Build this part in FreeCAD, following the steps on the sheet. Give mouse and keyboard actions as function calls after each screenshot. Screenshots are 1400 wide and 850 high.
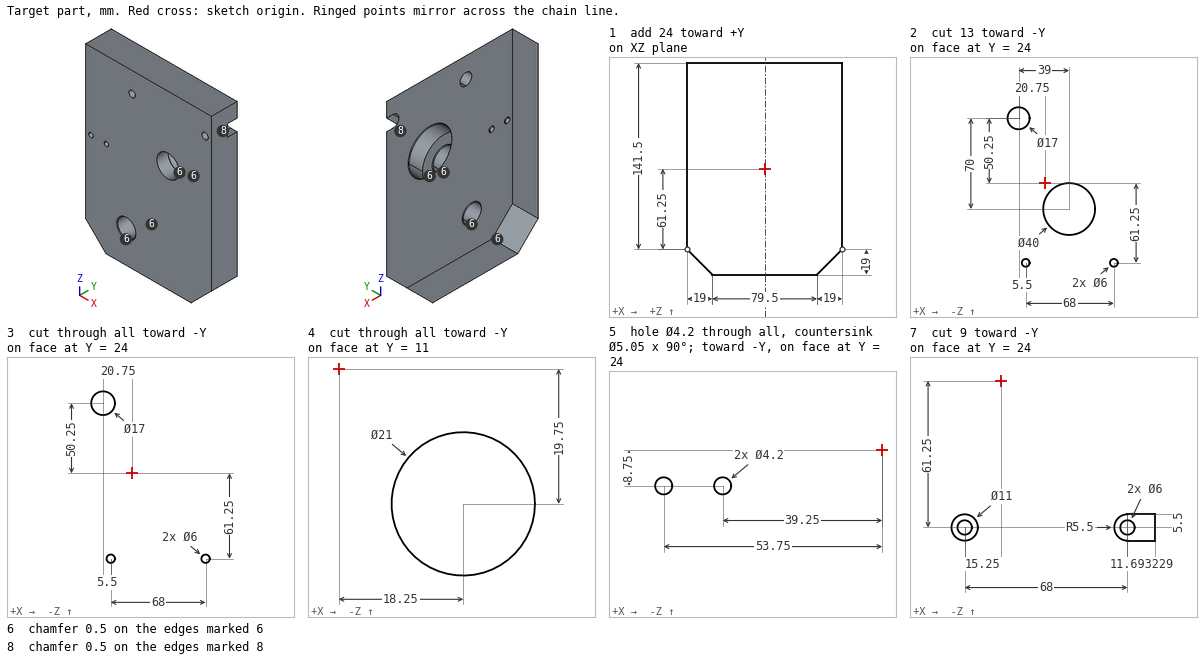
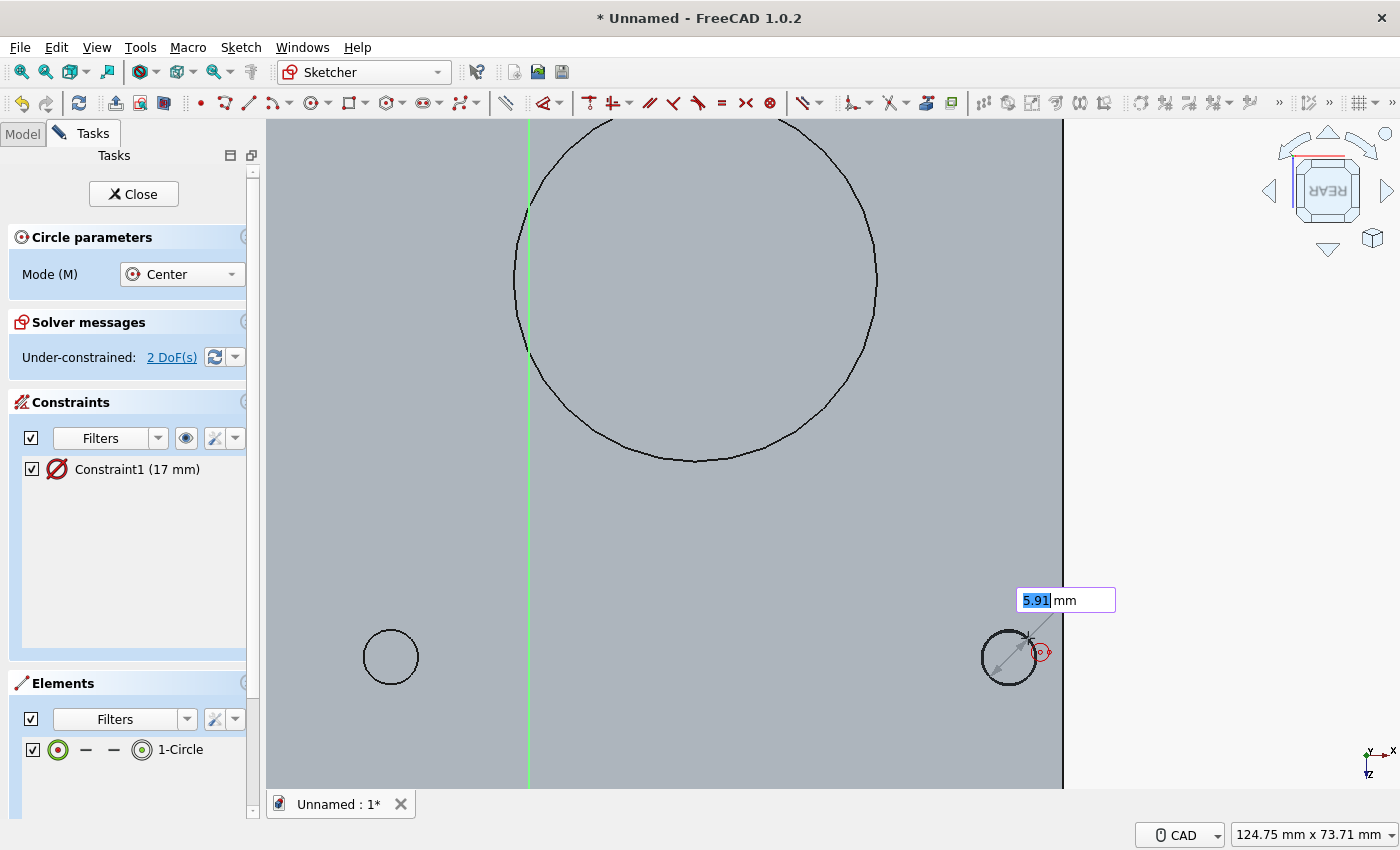
text(6)
key(Return)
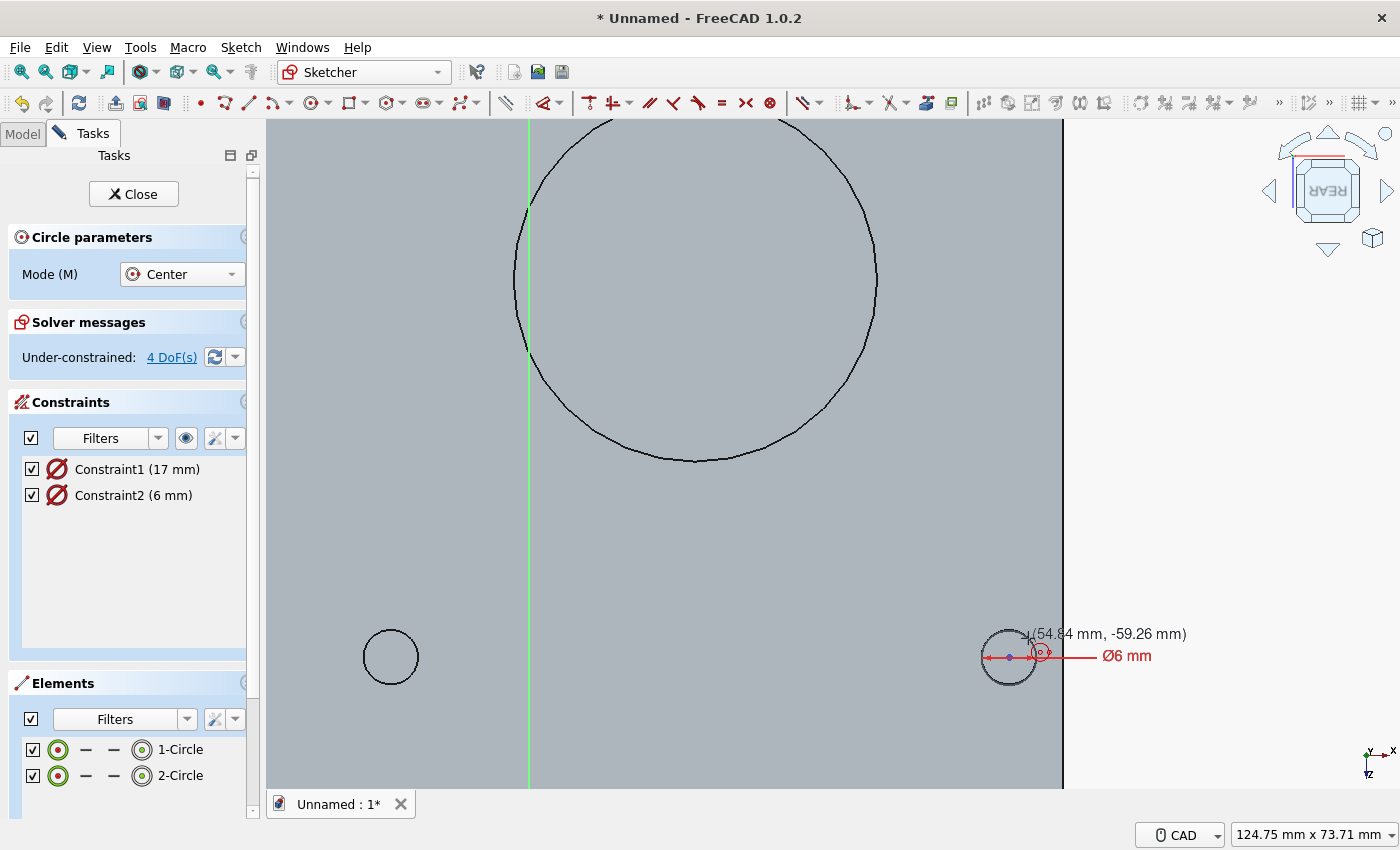
click(391, 657)
move(410, 638)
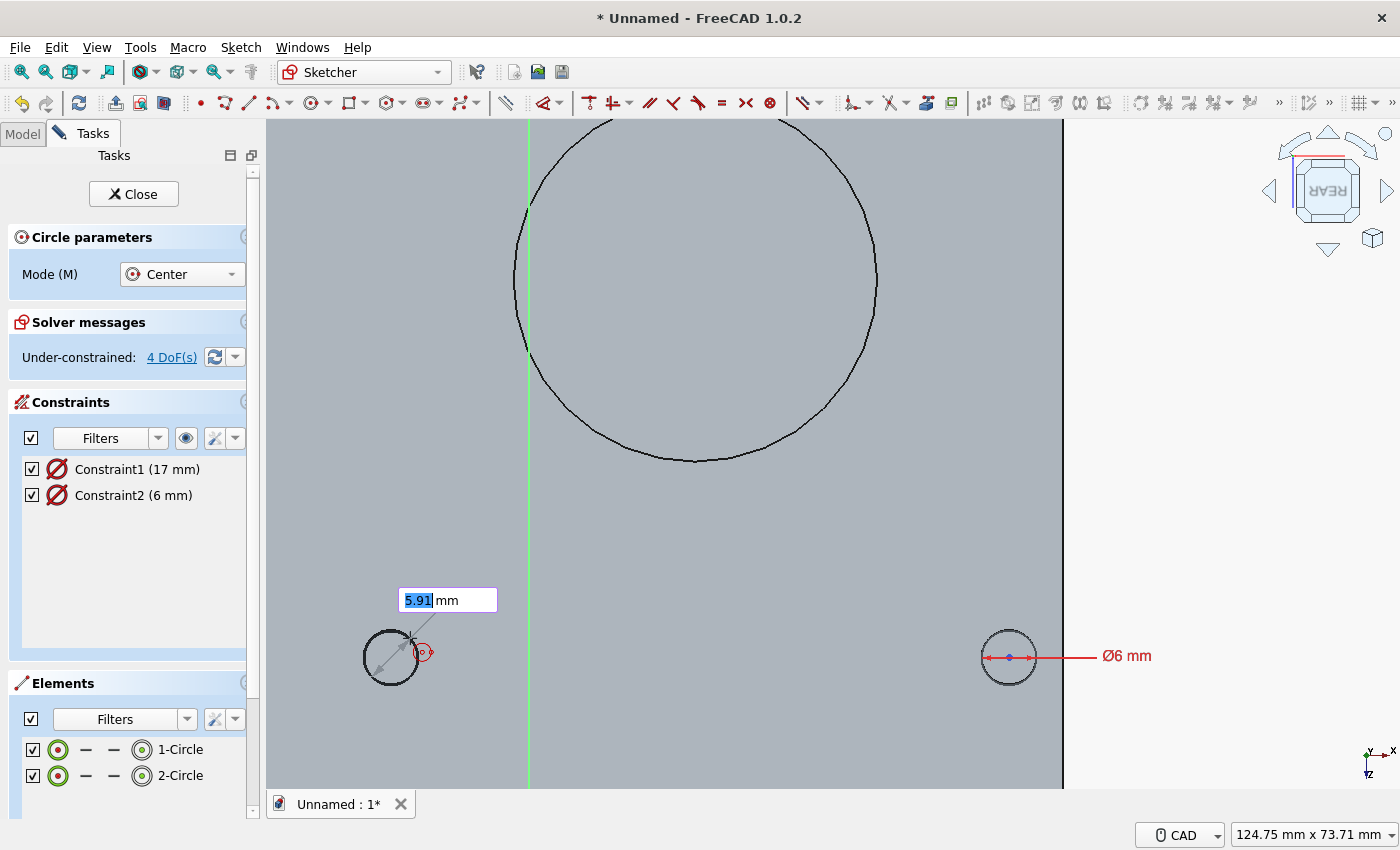
text(6)
key(Return)
key(Escape)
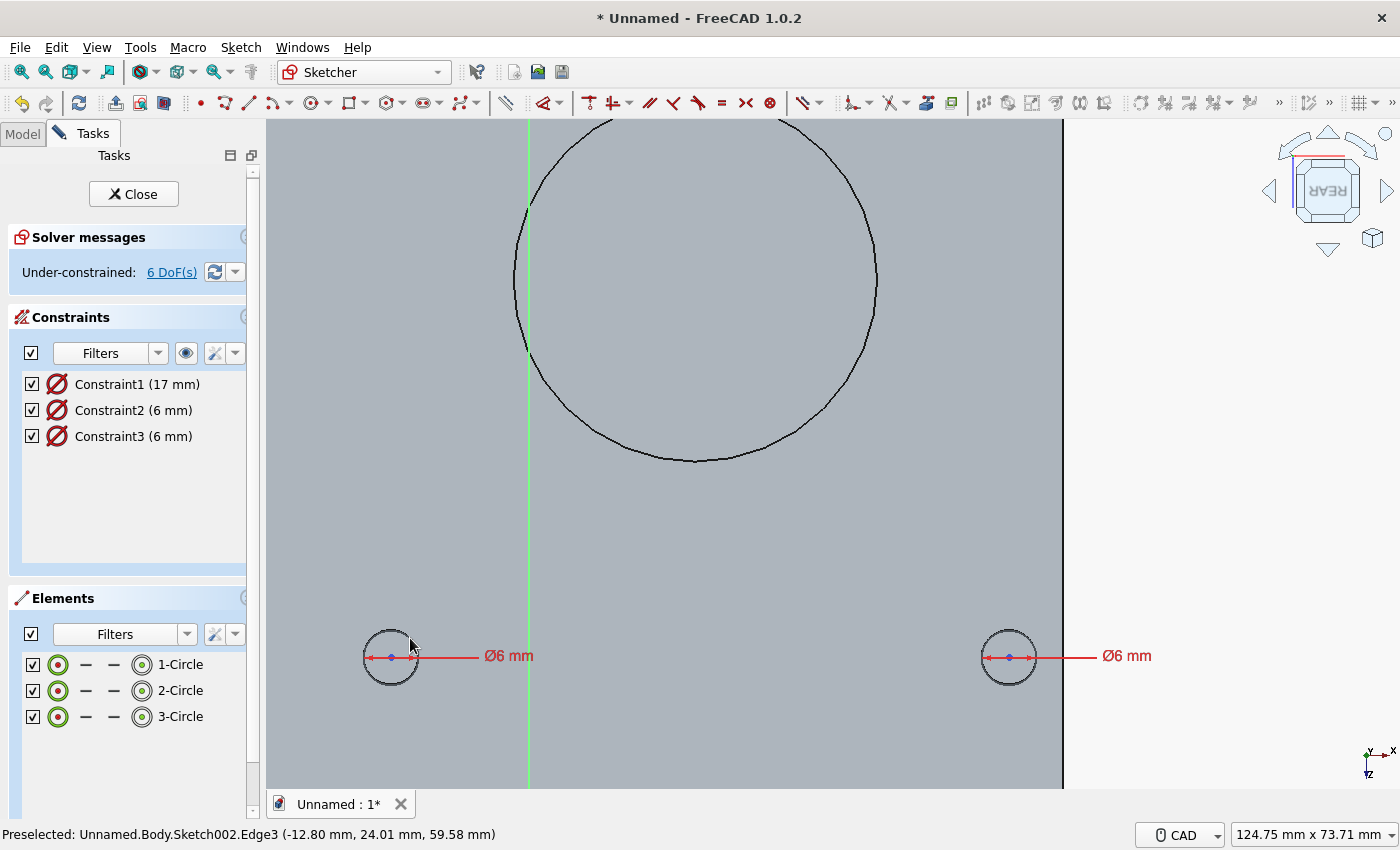
click(1009, 658)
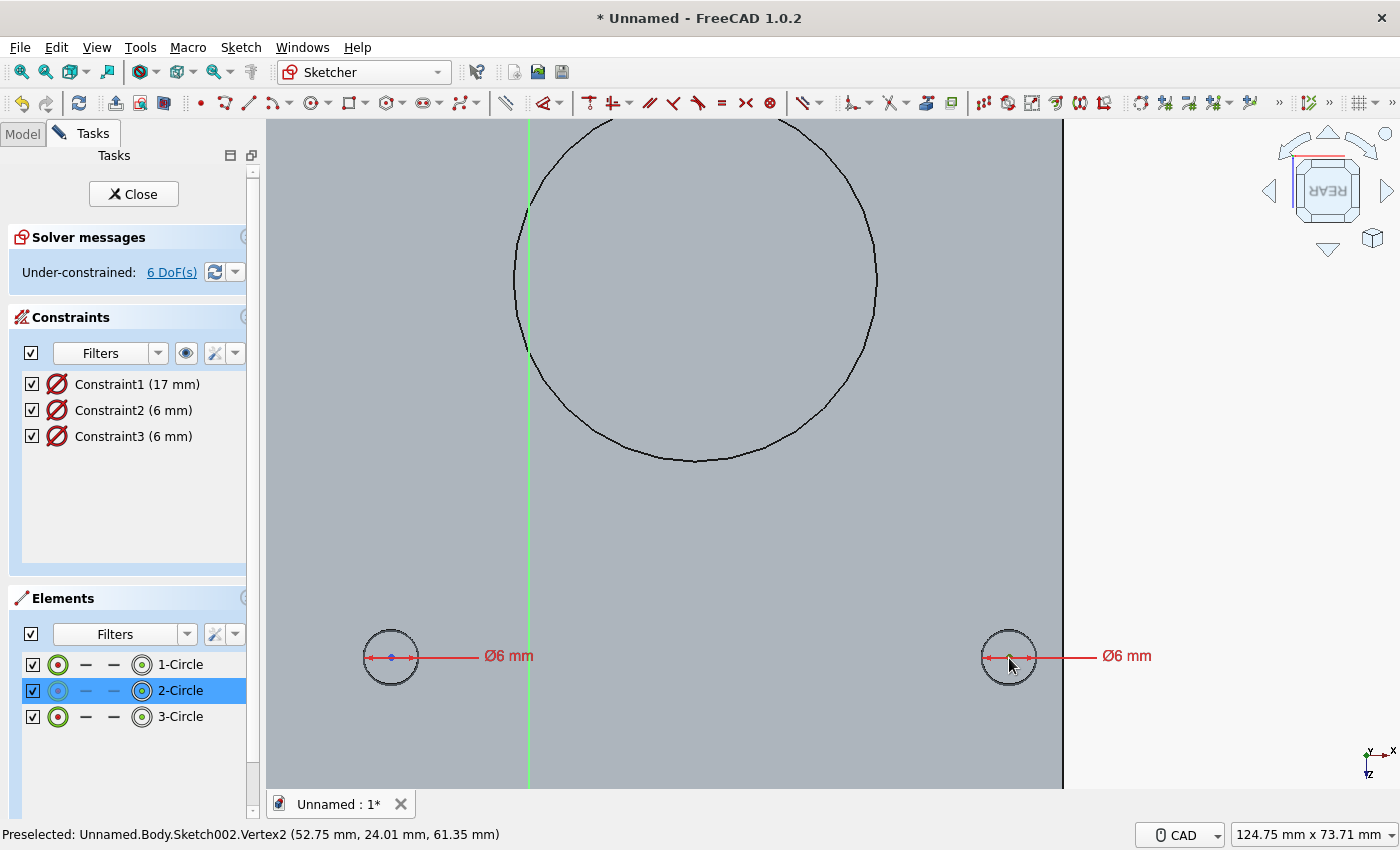
click(391, 658)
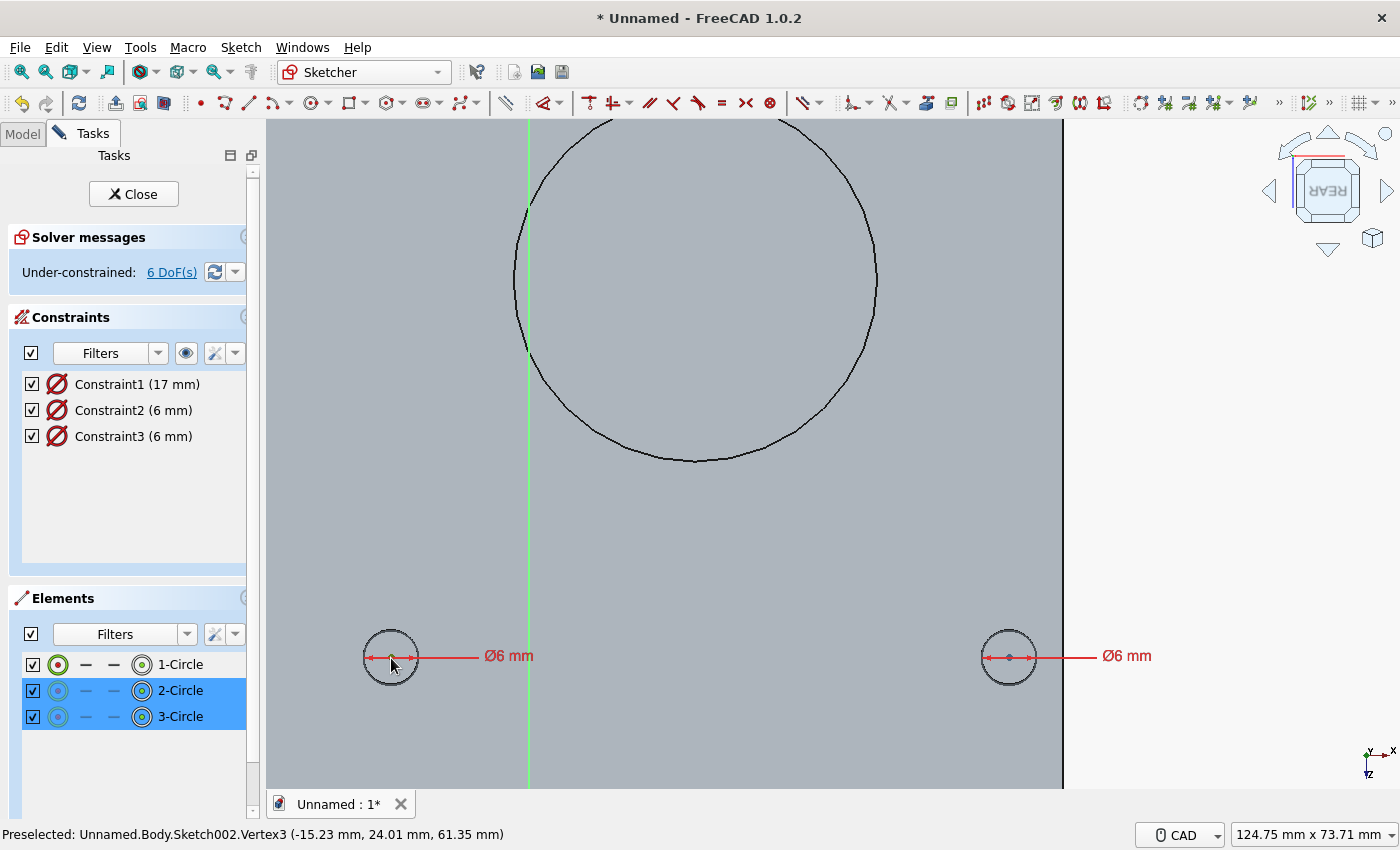
key(h)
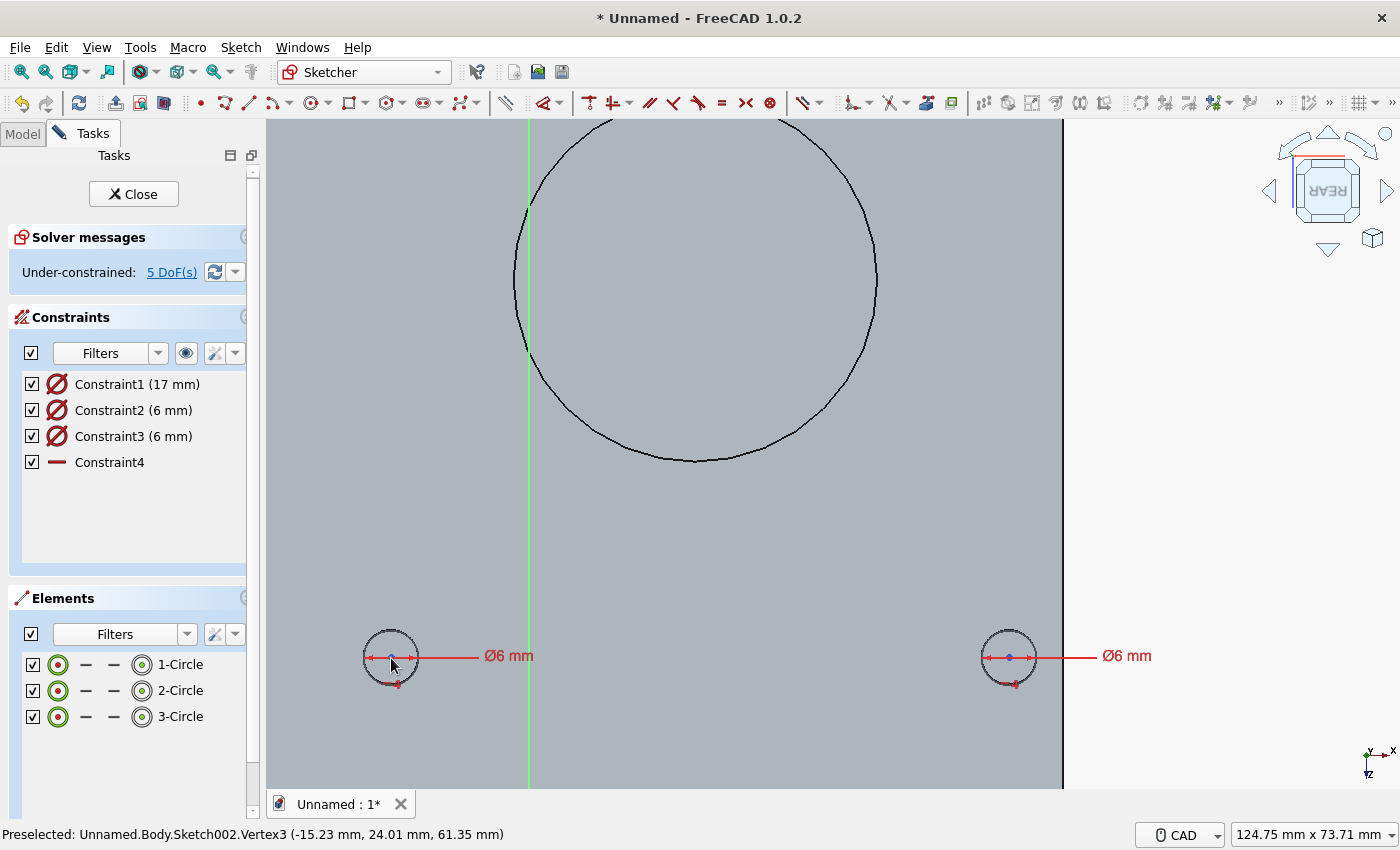
key(d)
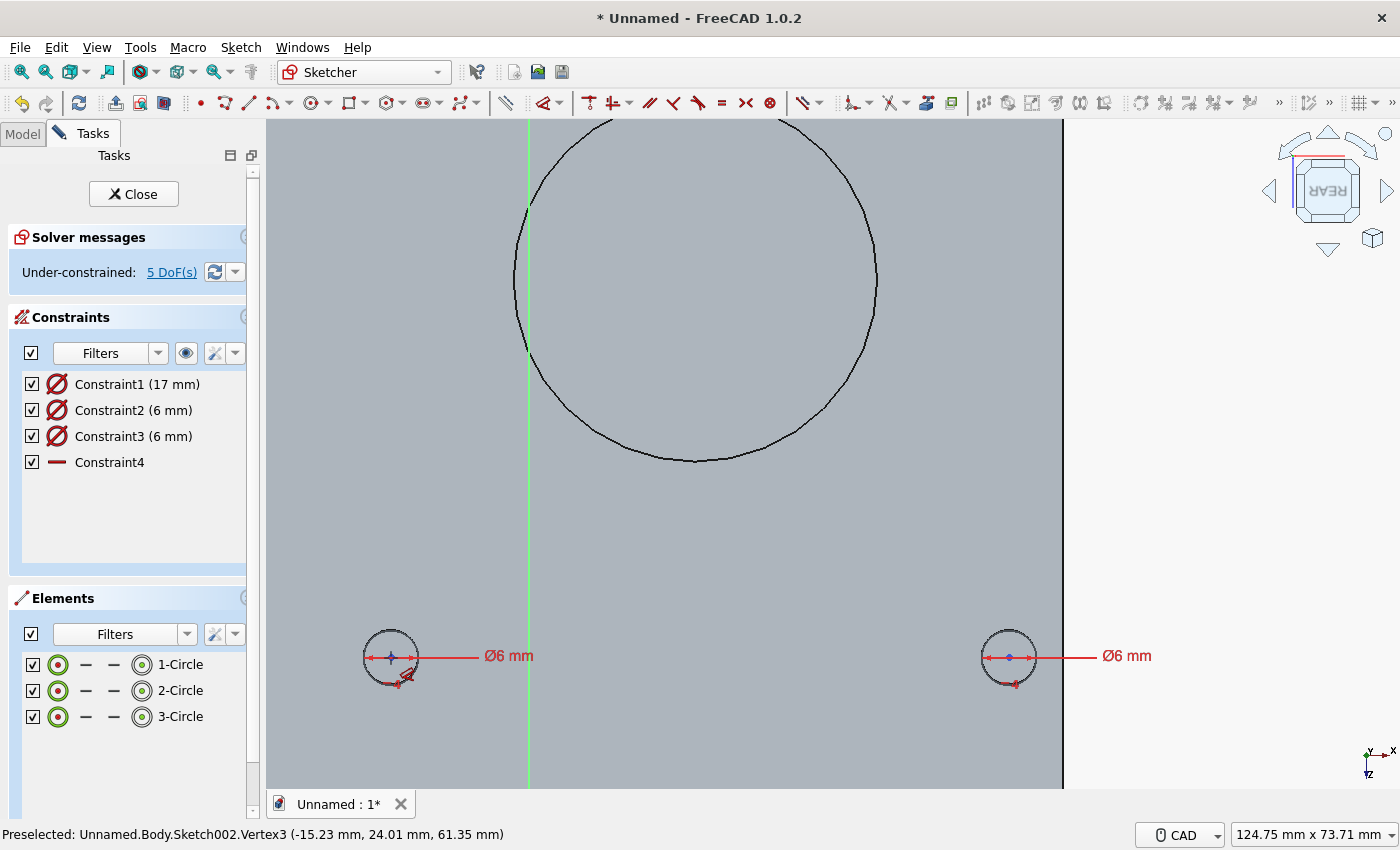
click(1009, 658)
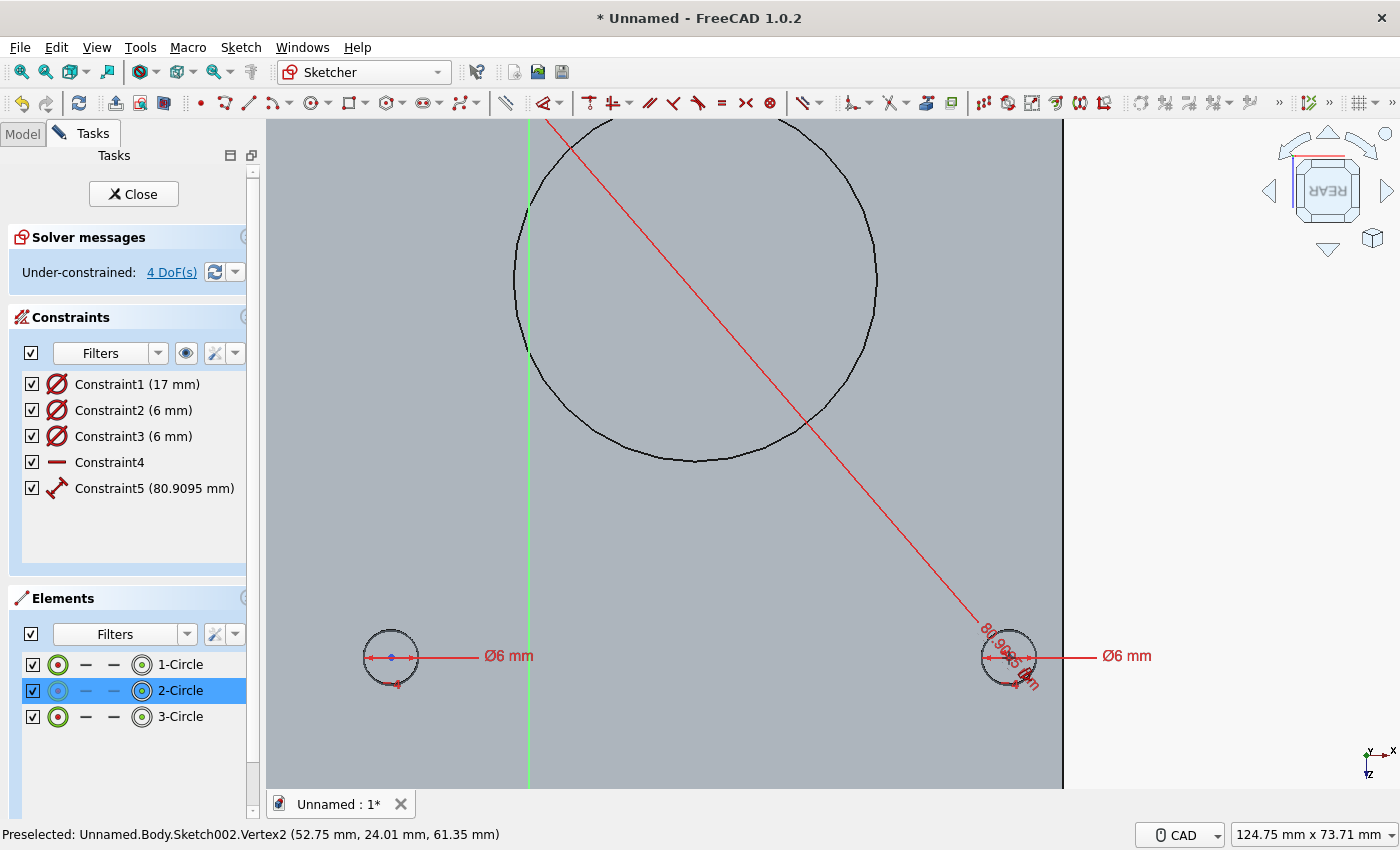
click(391, 658)
click(700, 692)